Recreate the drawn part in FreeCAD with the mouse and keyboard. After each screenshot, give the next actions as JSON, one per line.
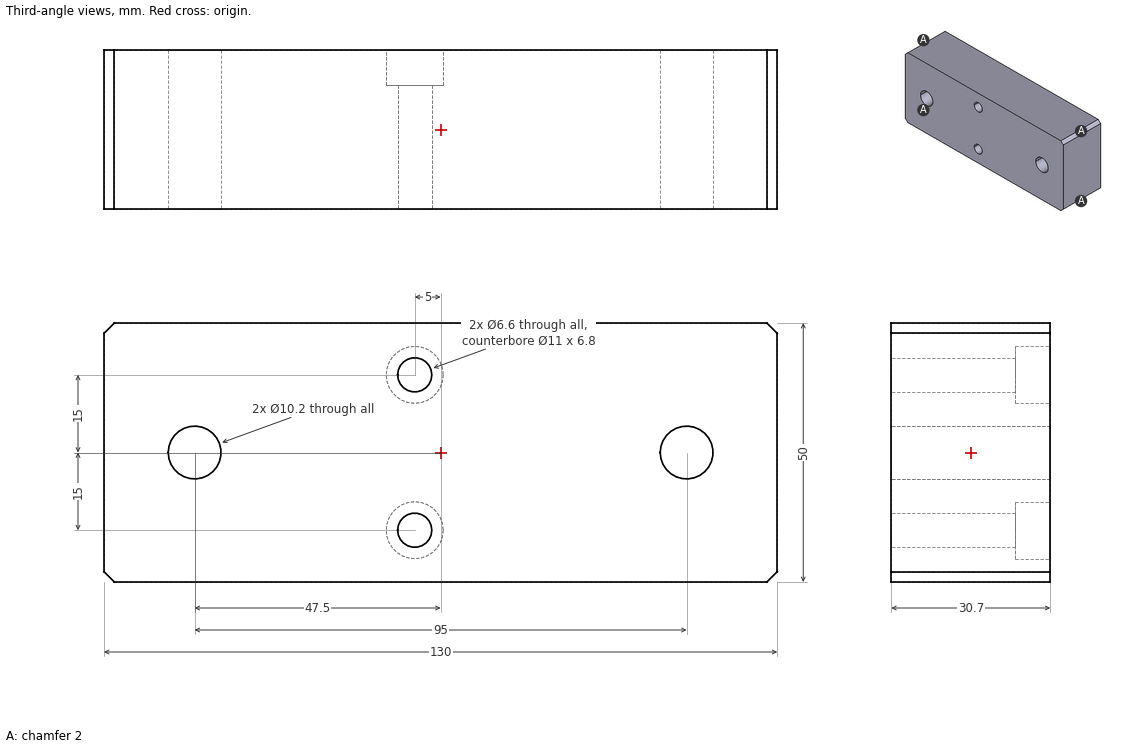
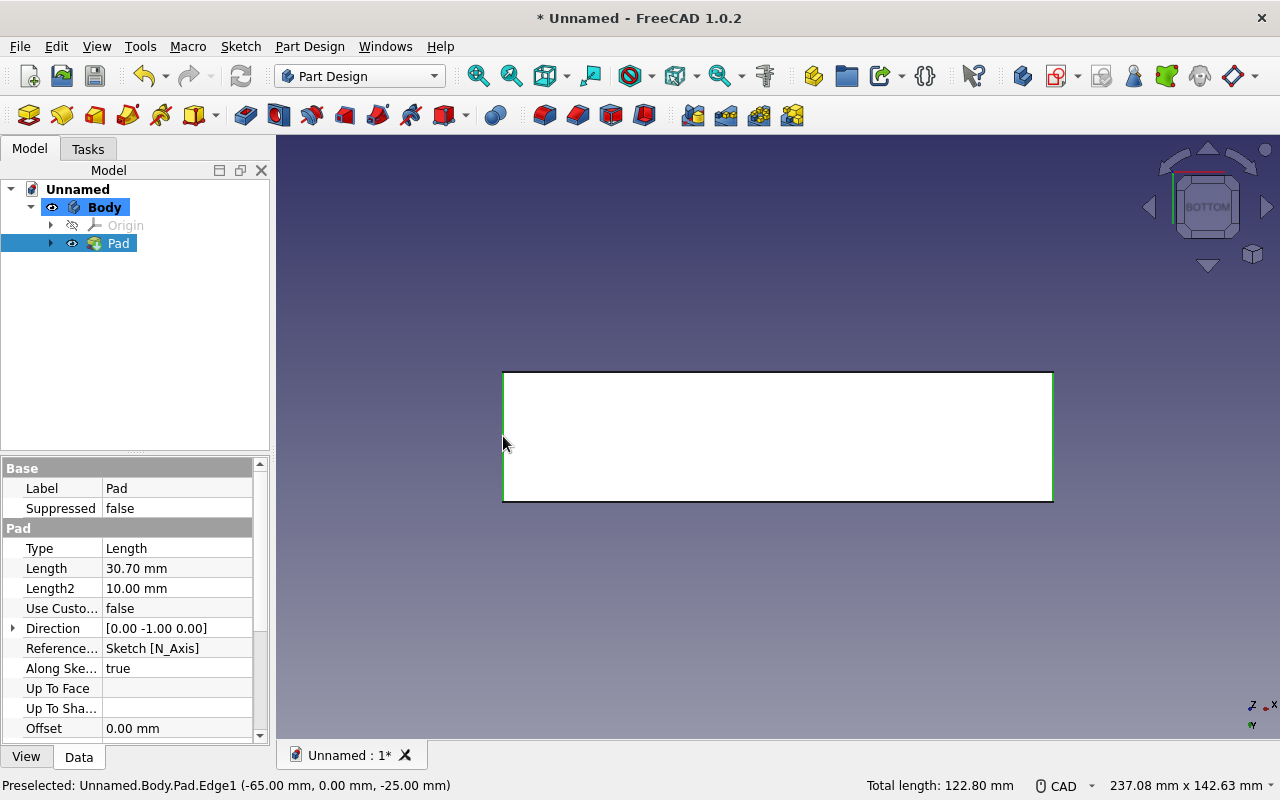
{"action": "left_click", "coordinate": [578, 116]}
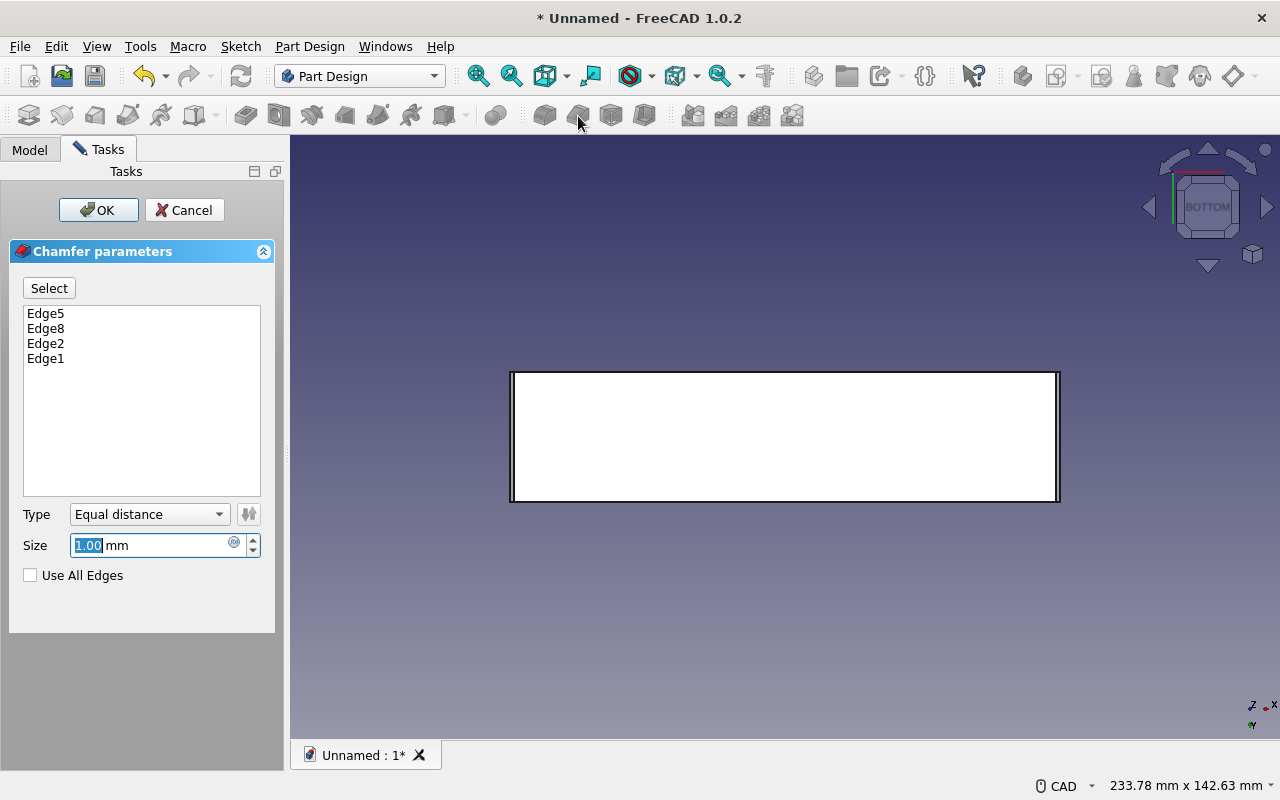
{"action": "type", "text": "2"}
{"action": "key", "text": "Tab"}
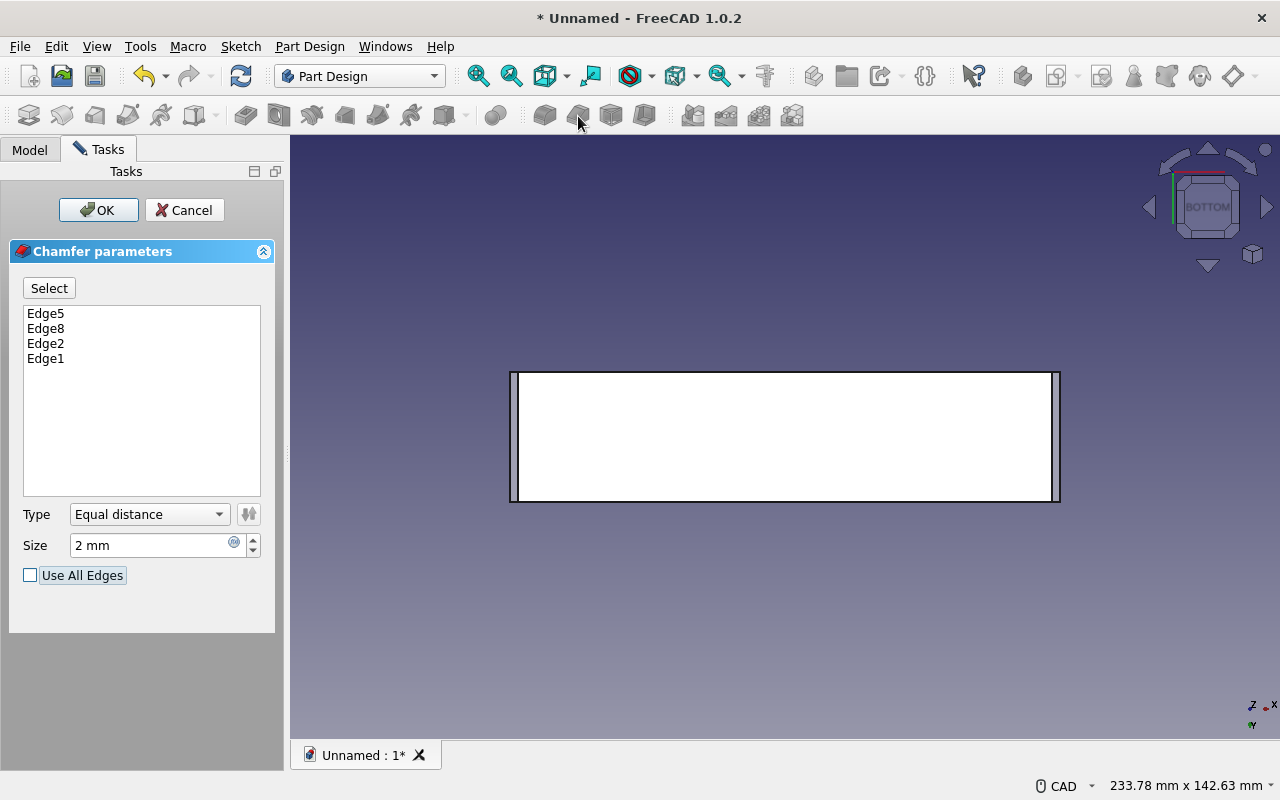
{"action": "left_click", "coordinate": [99, 210]}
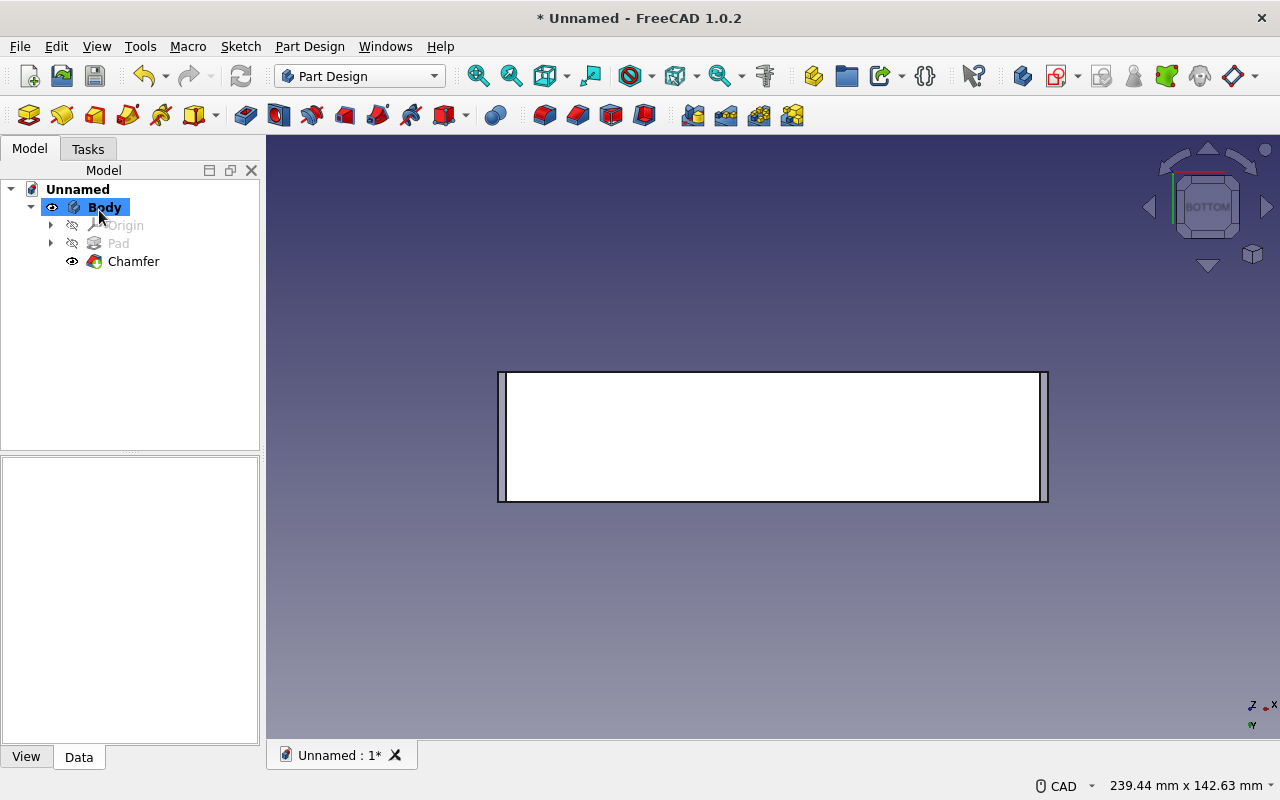
{"action": "key", "text": "4"}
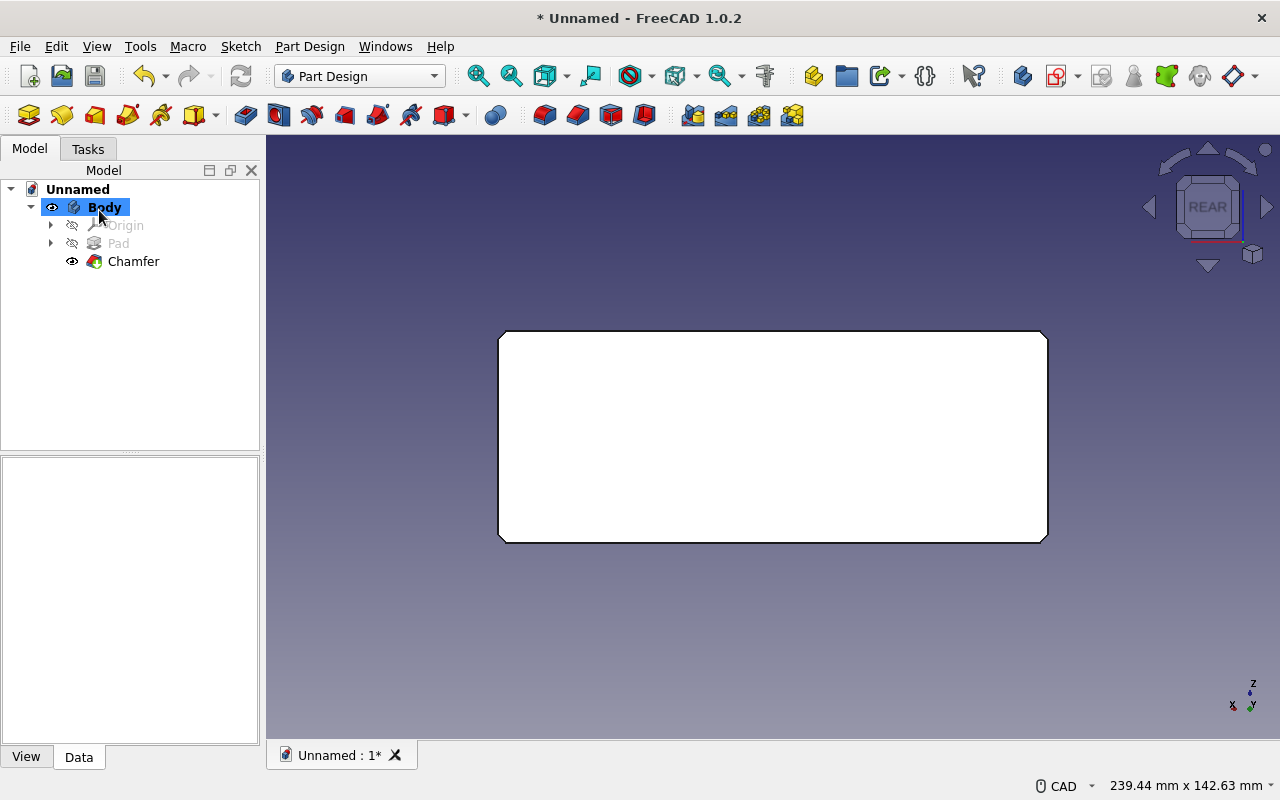
{"action": "left_click", "coordinate": [616, 436]}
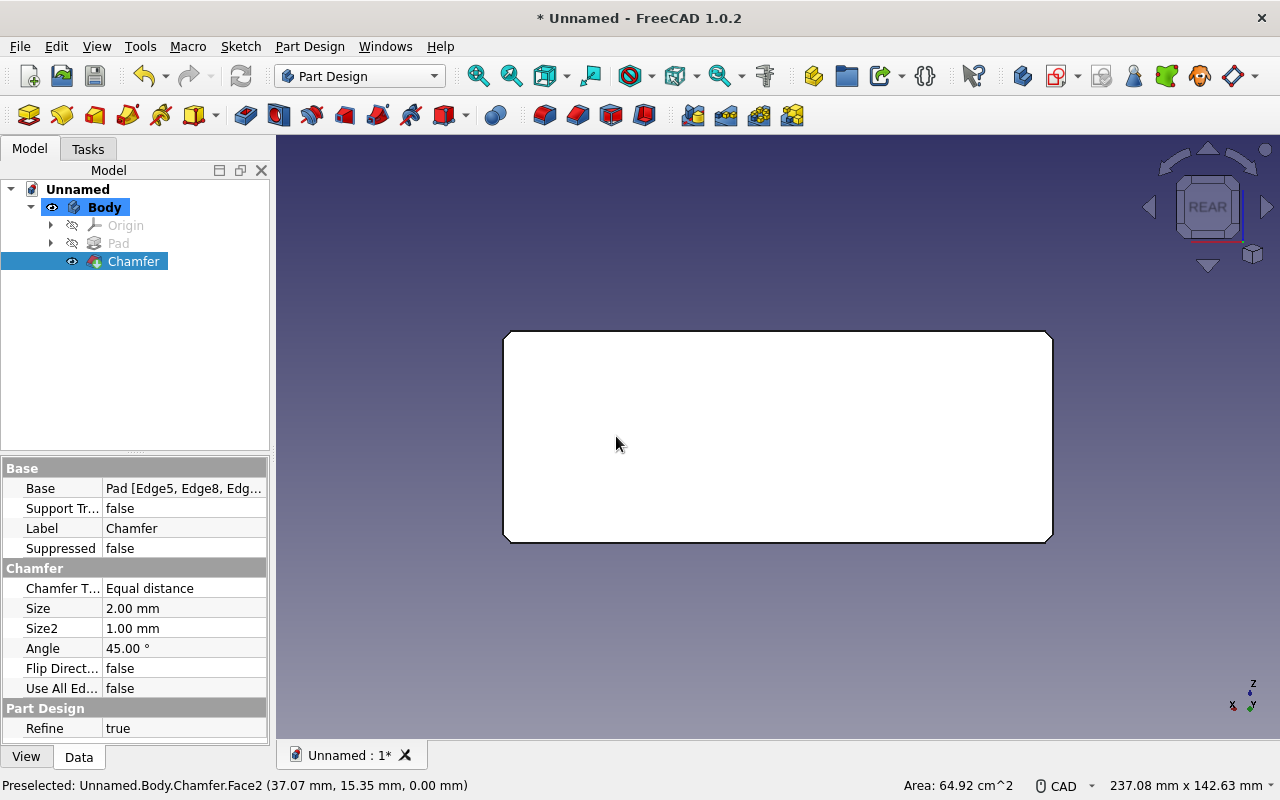
{"action": "left_click", "coordinate": [1056, 76]}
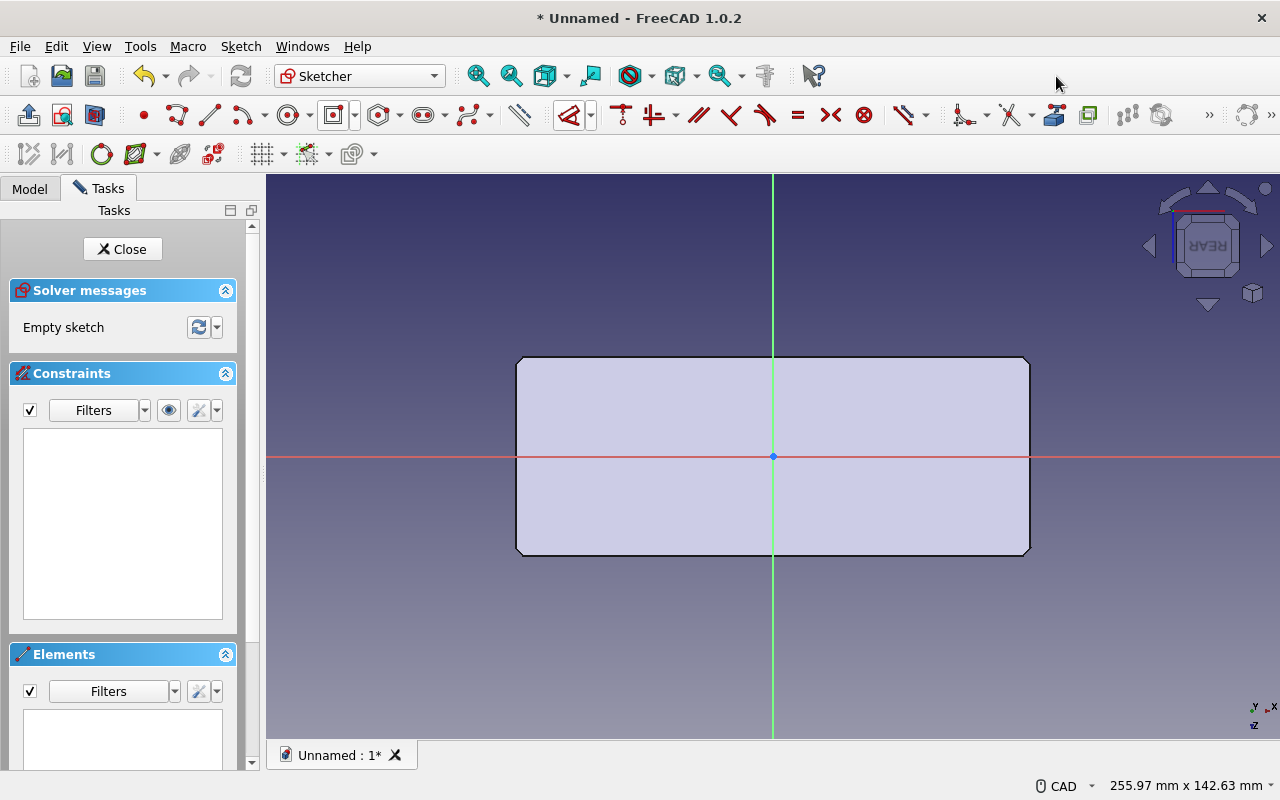
{"action": "scroll", "coordinate": [912, 457], "scroll_direction": "up", "scroll_amount": 2}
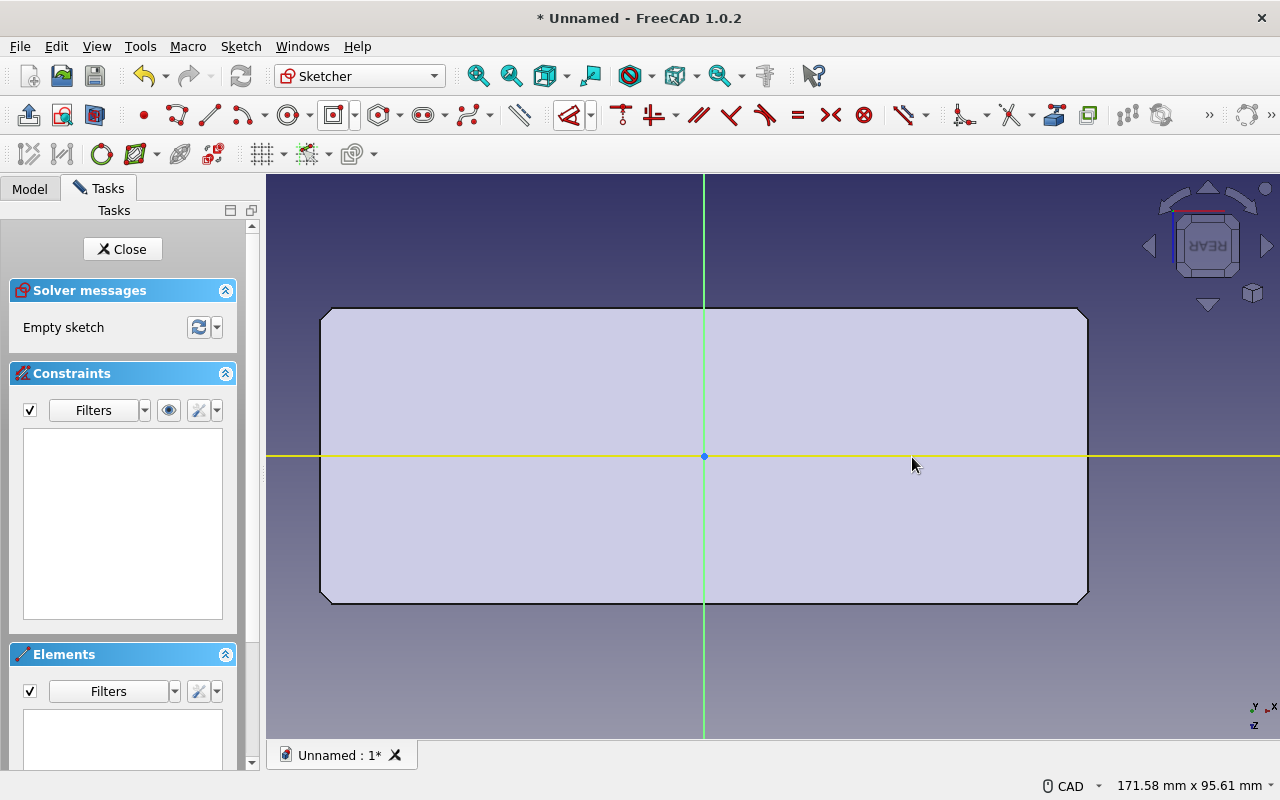
{"action": "left_click", "coordinate": [288, 116]}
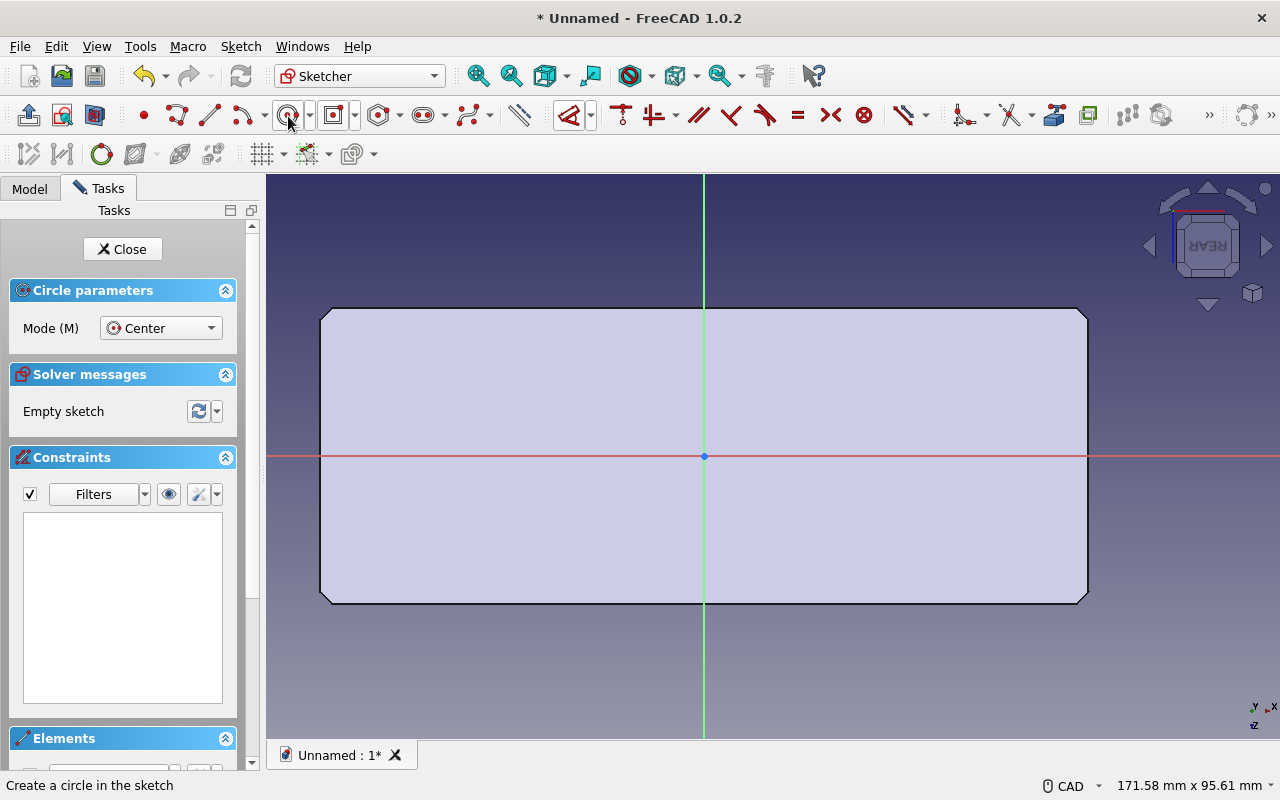
{"action": "left_click", "coordinate": [424, 456]}
{"action": "left_click", "coordinate": [445, 435]}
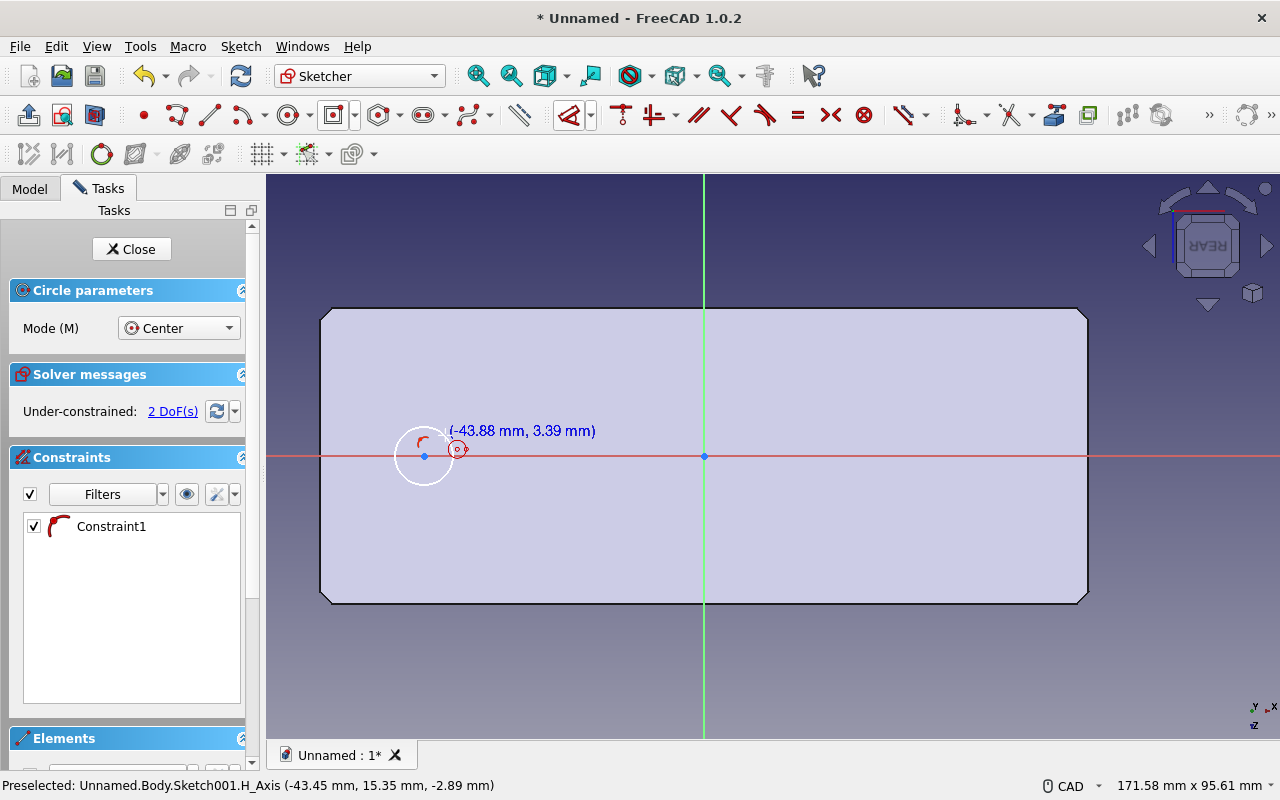
{"action": "left_click", "coordinate": [985, 456]}
{"action": "left_click", "coordinate": [1006, 435]}
{"action": "key", "text": "Escape"}